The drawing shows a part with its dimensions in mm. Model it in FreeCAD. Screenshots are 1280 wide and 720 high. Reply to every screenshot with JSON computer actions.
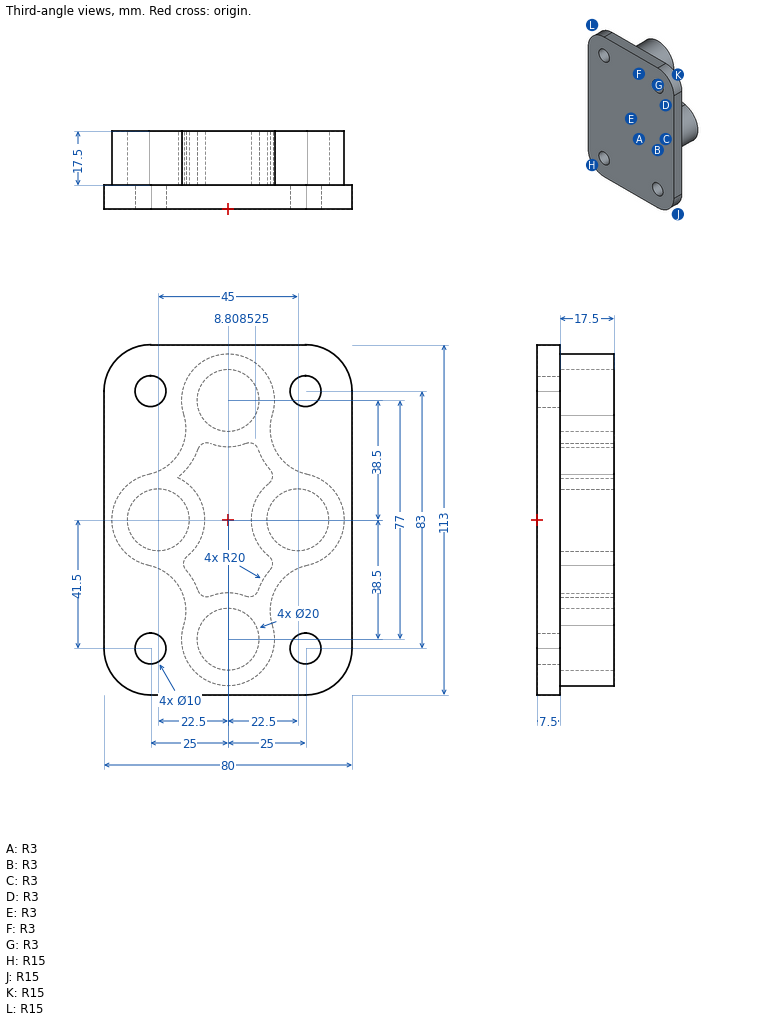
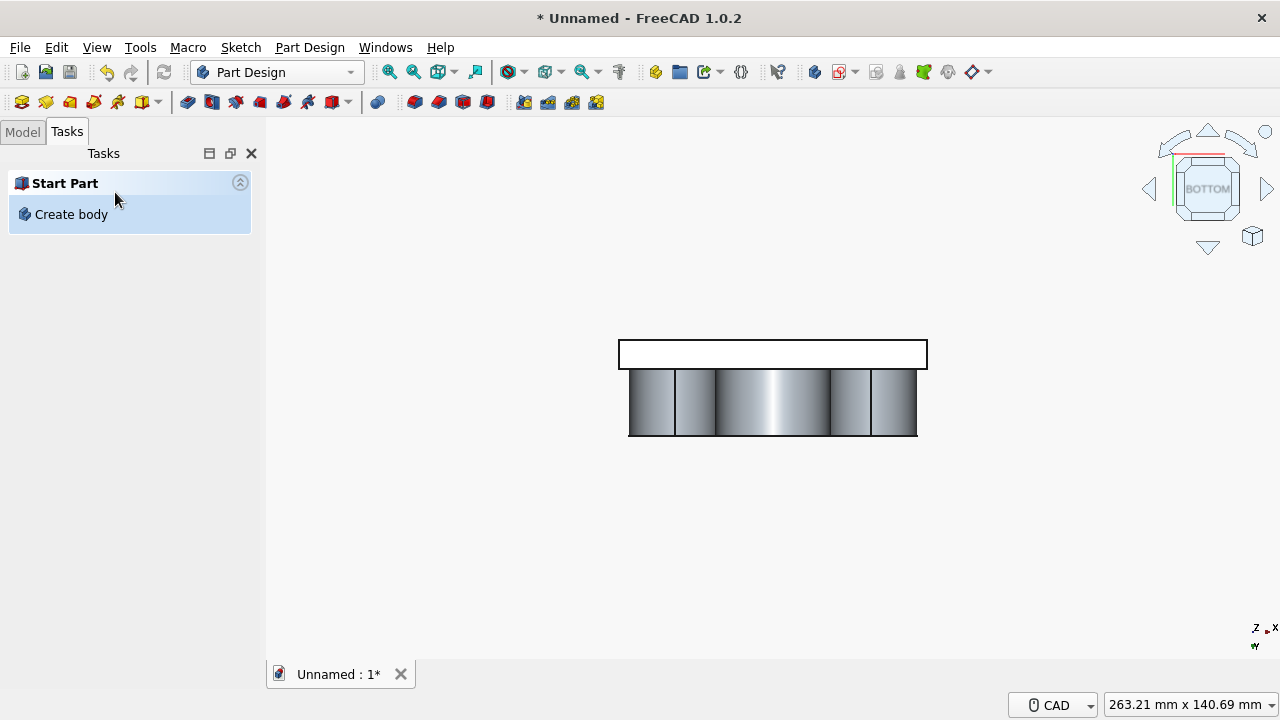
{"action": "left_click", "coordinate": [619, 353]}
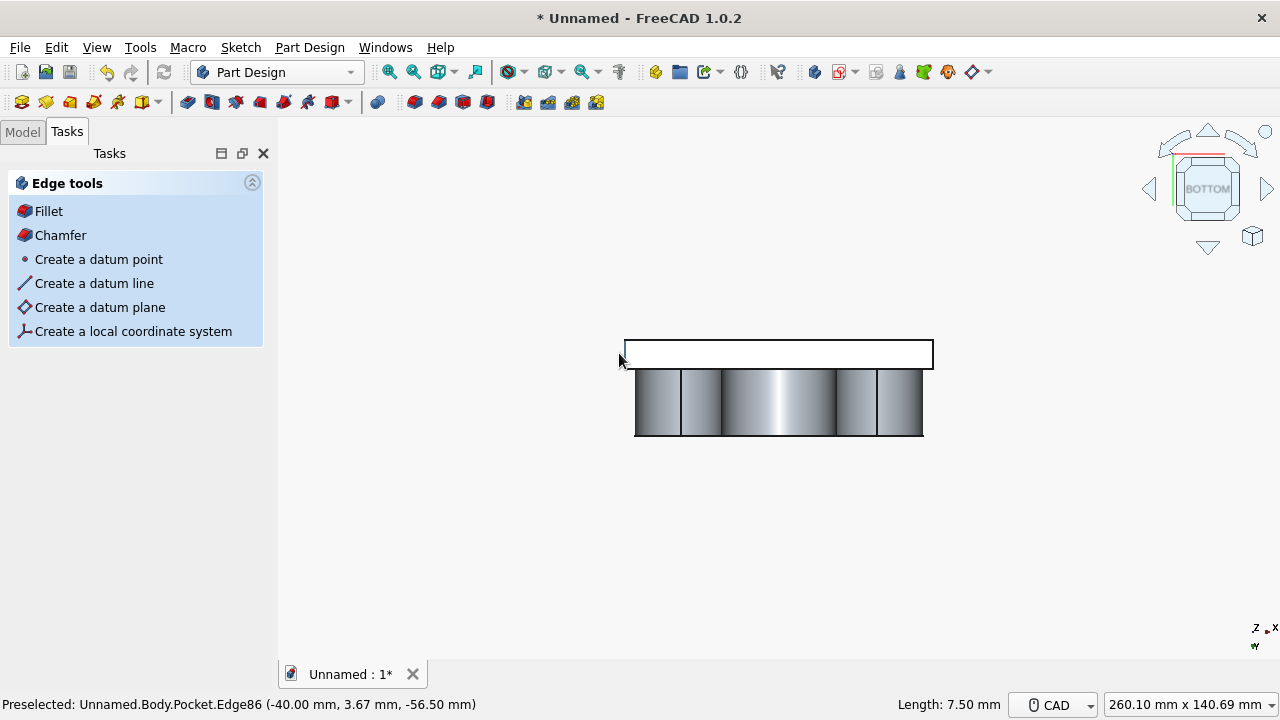
{"action": "left_click", "coordinate": [416, 102]}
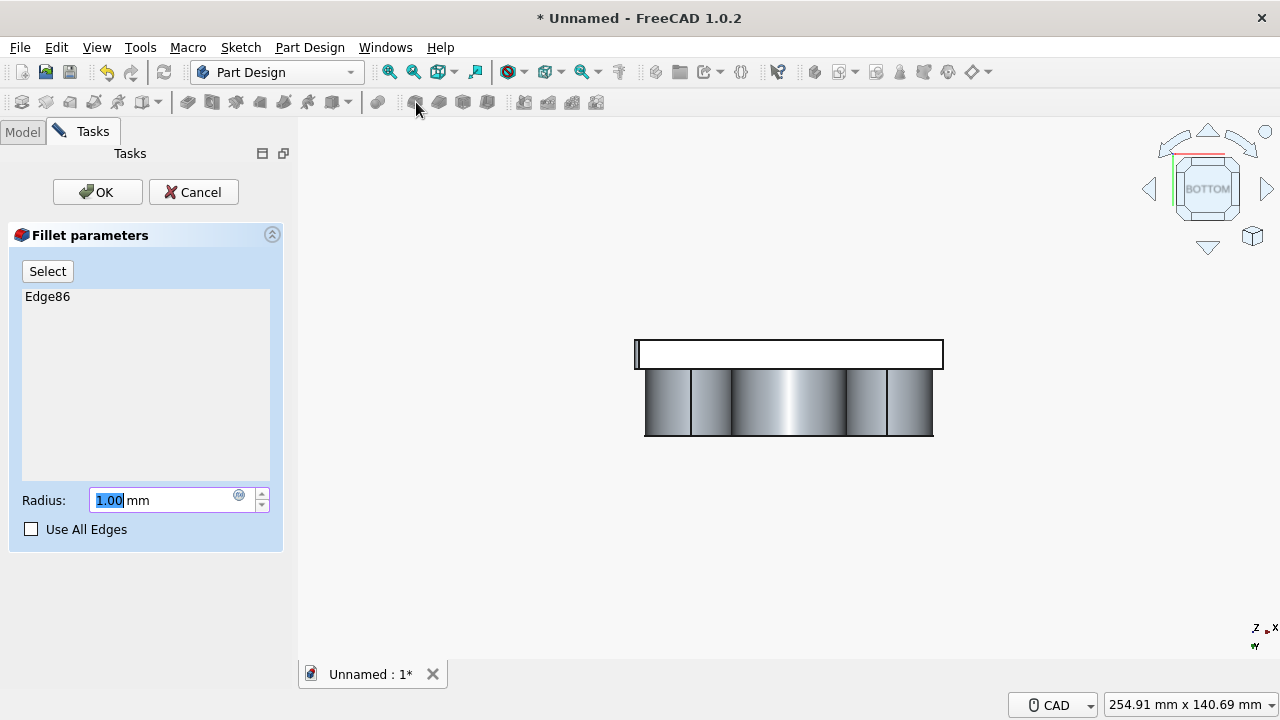
{"action": "type", "text": "15"}
{"action": "key", "text": "Tab"}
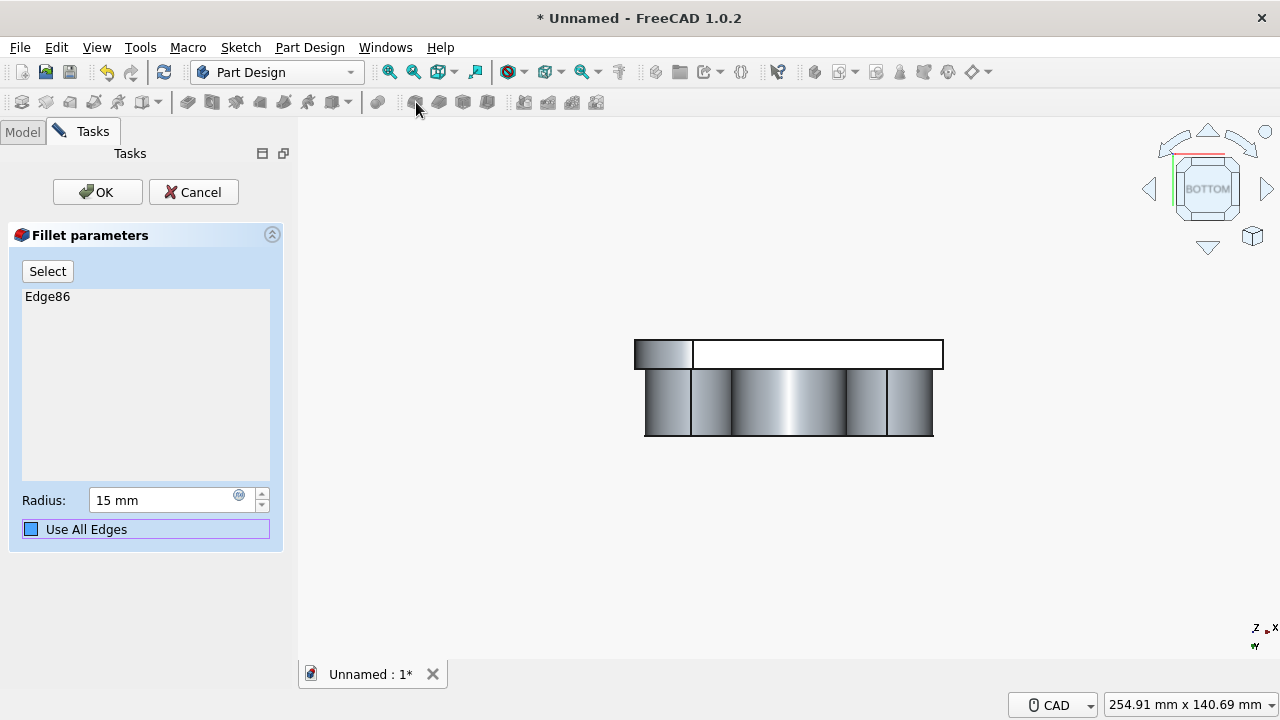
{"action": "left_click", "coordinate": [98, 192]}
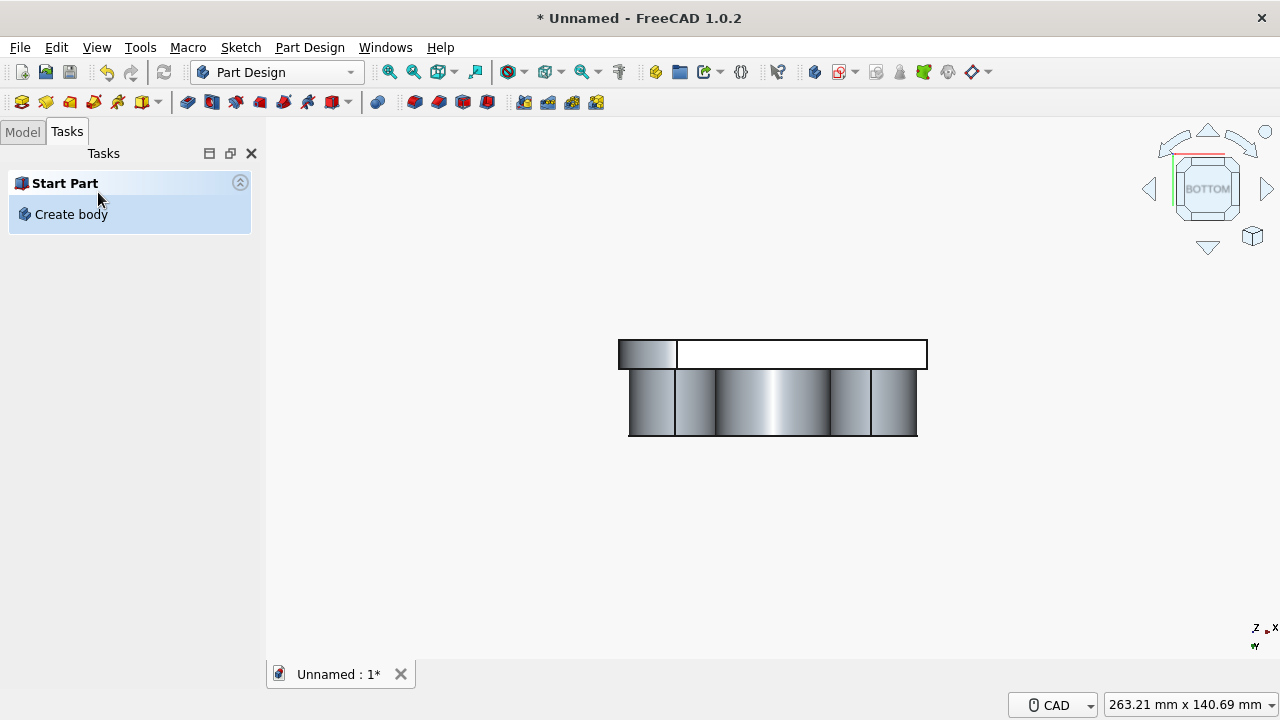
{"action": "key", "text": "v f"}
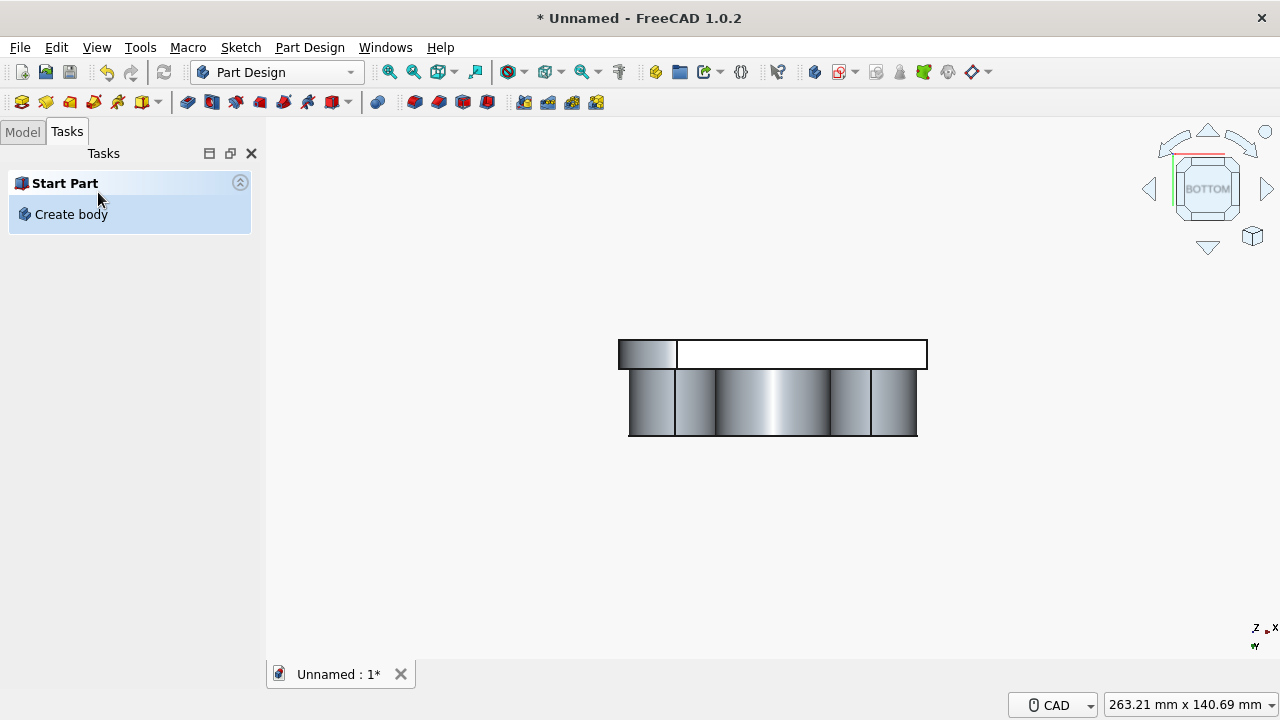
{"action": "left_click", "coordinate": [927, 353]}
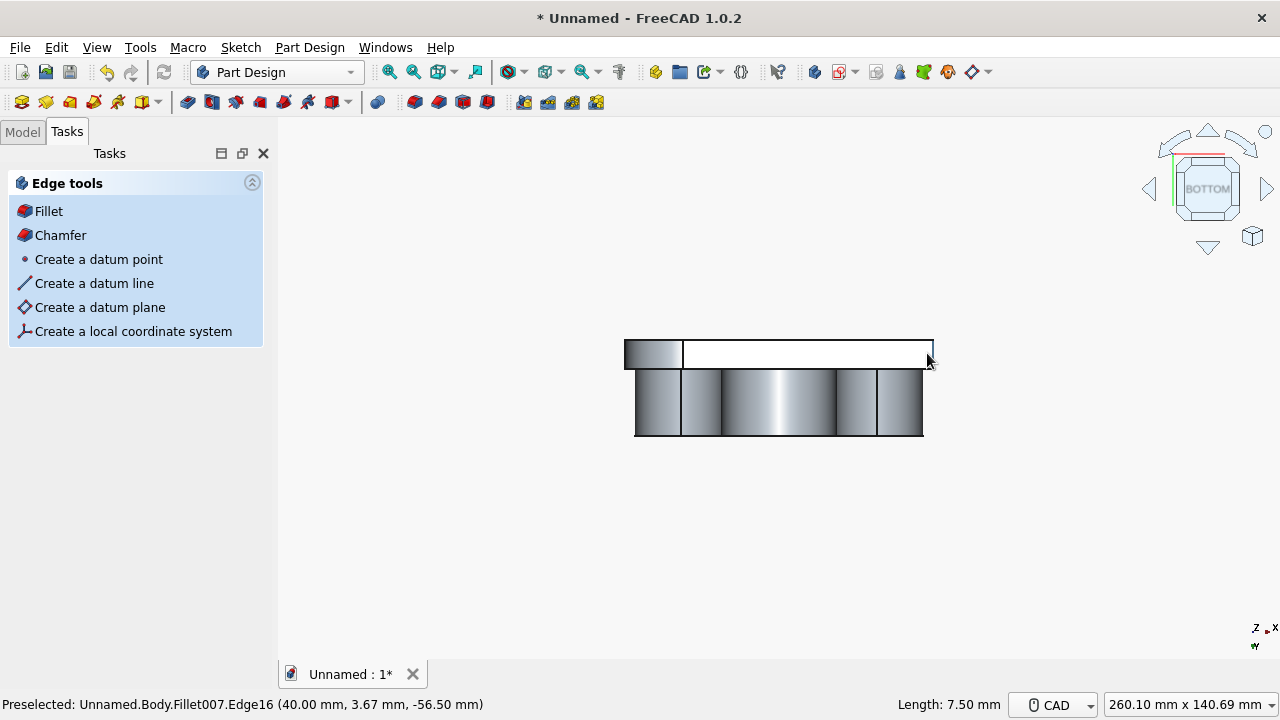
{"action": "left_click", "coordinate": [416, 102]}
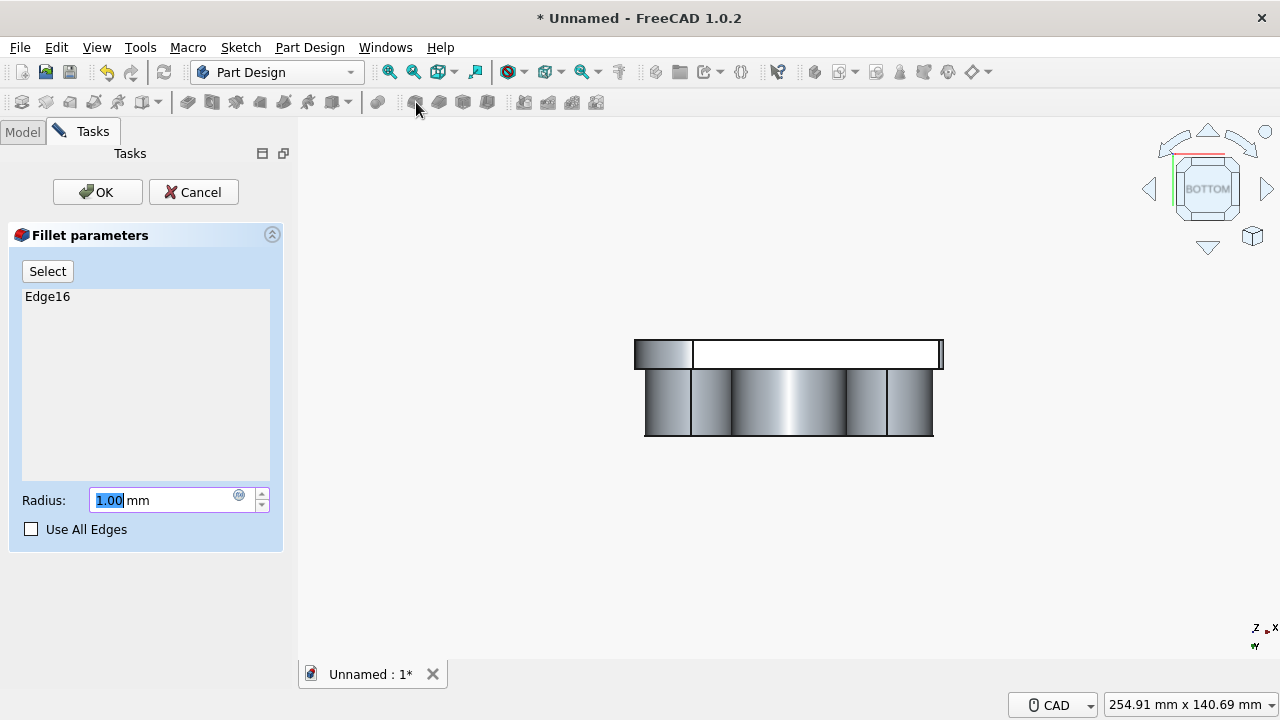
{"action": "type", "text": "15"}
{"action": "key", "text": "Tab"}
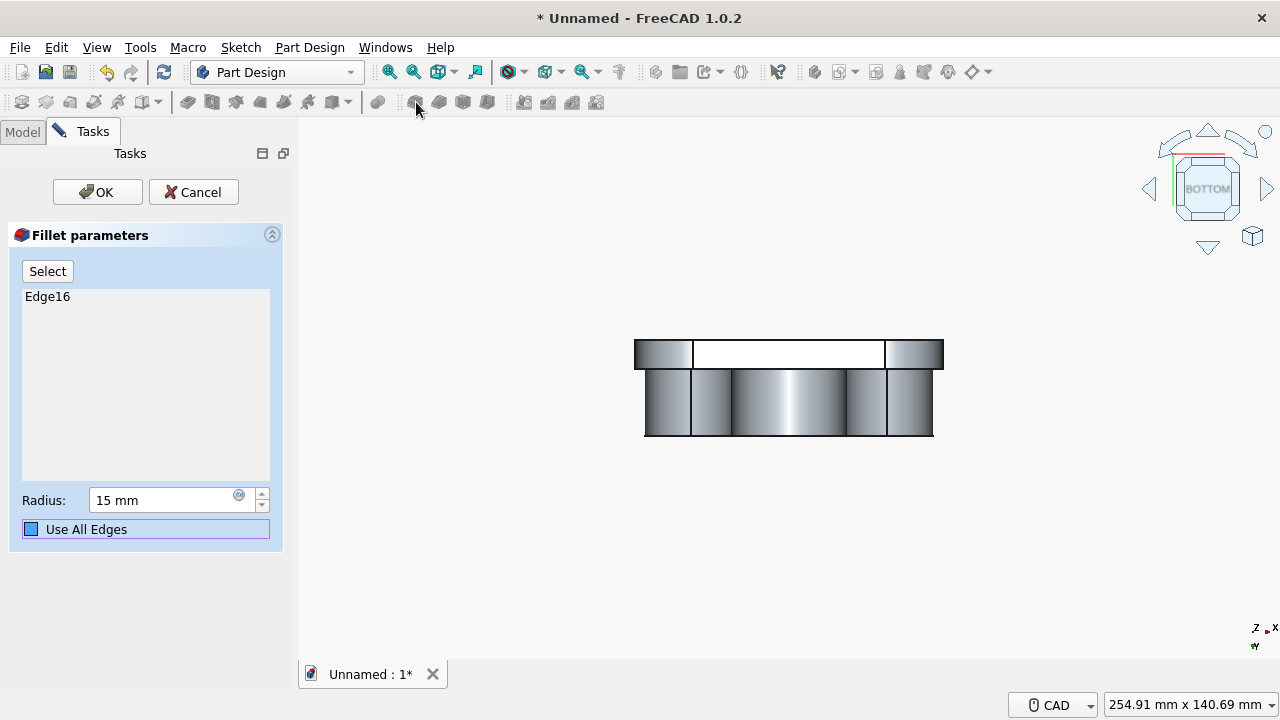
{"action": "left_click", "coordinate": [98, 192]}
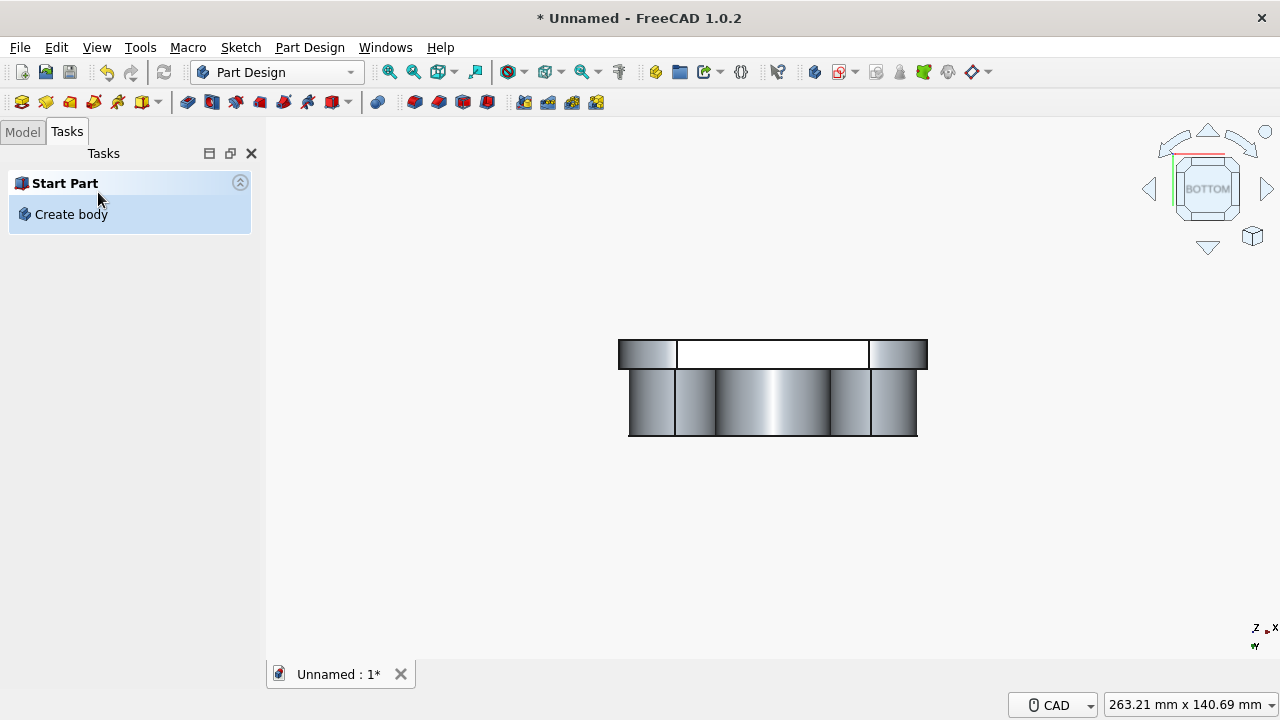
{"action": "key", "text": "v f"}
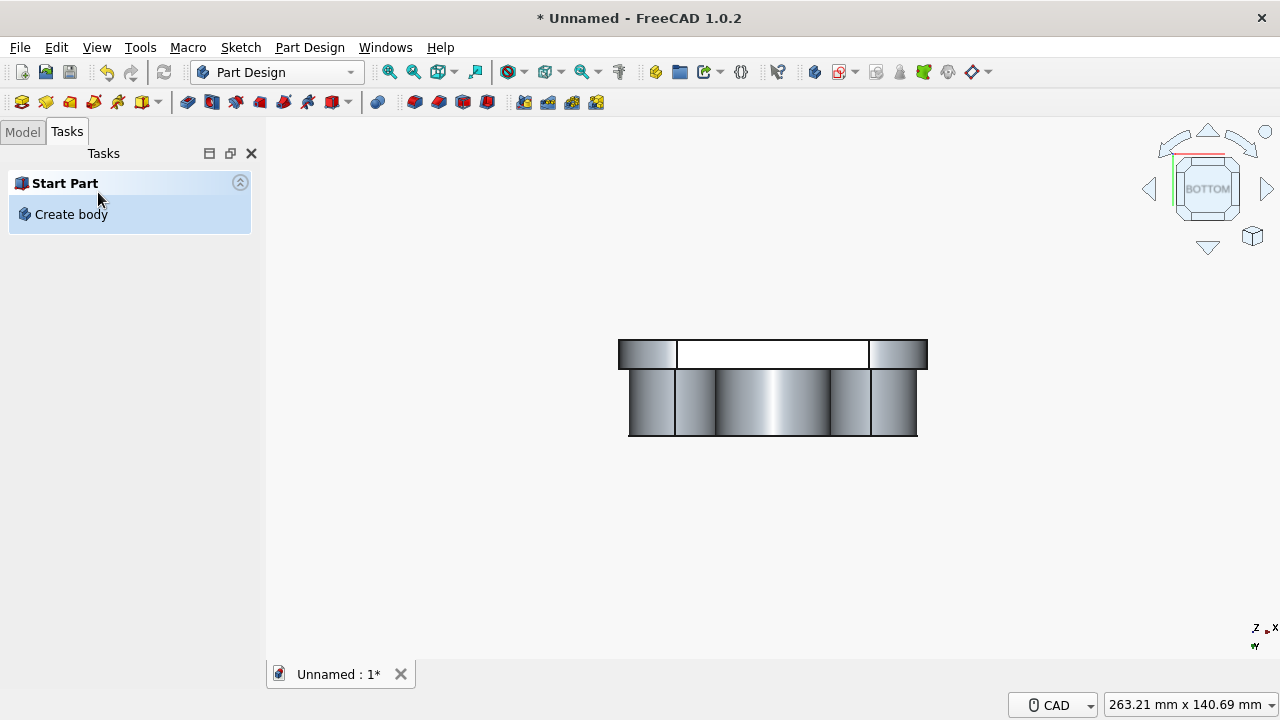
{"action": "key", "text": "0"}